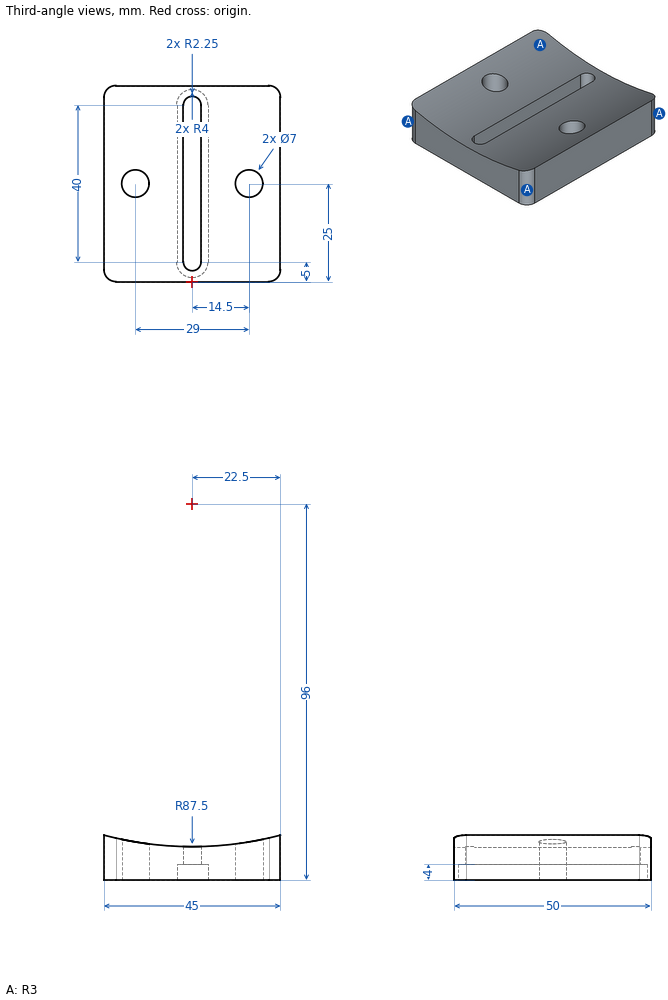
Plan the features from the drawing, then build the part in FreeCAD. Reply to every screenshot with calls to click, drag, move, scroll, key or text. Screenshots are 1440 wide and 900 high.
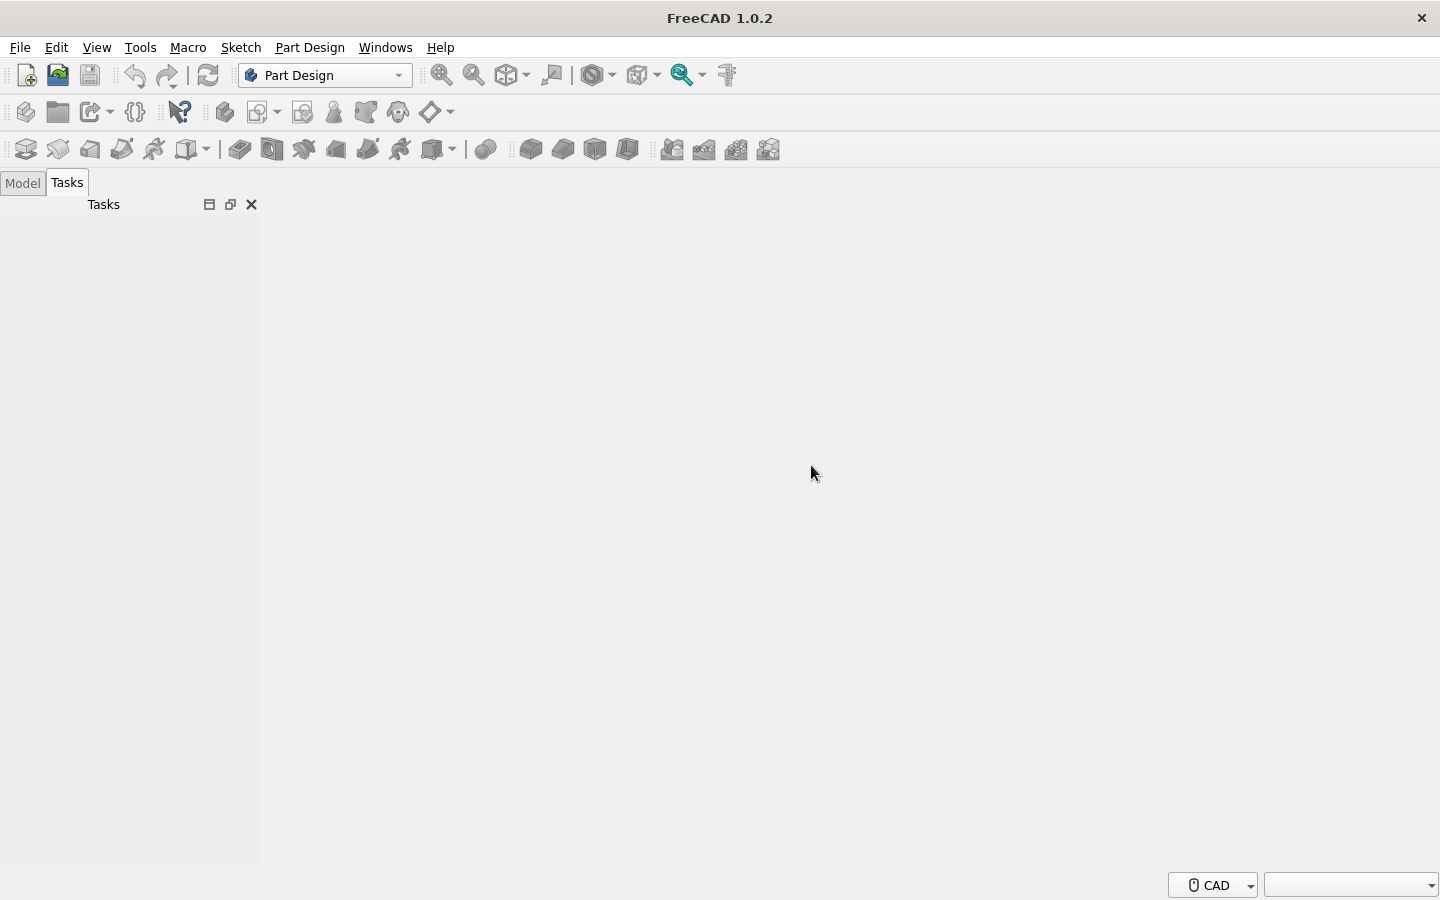
click(26, 76)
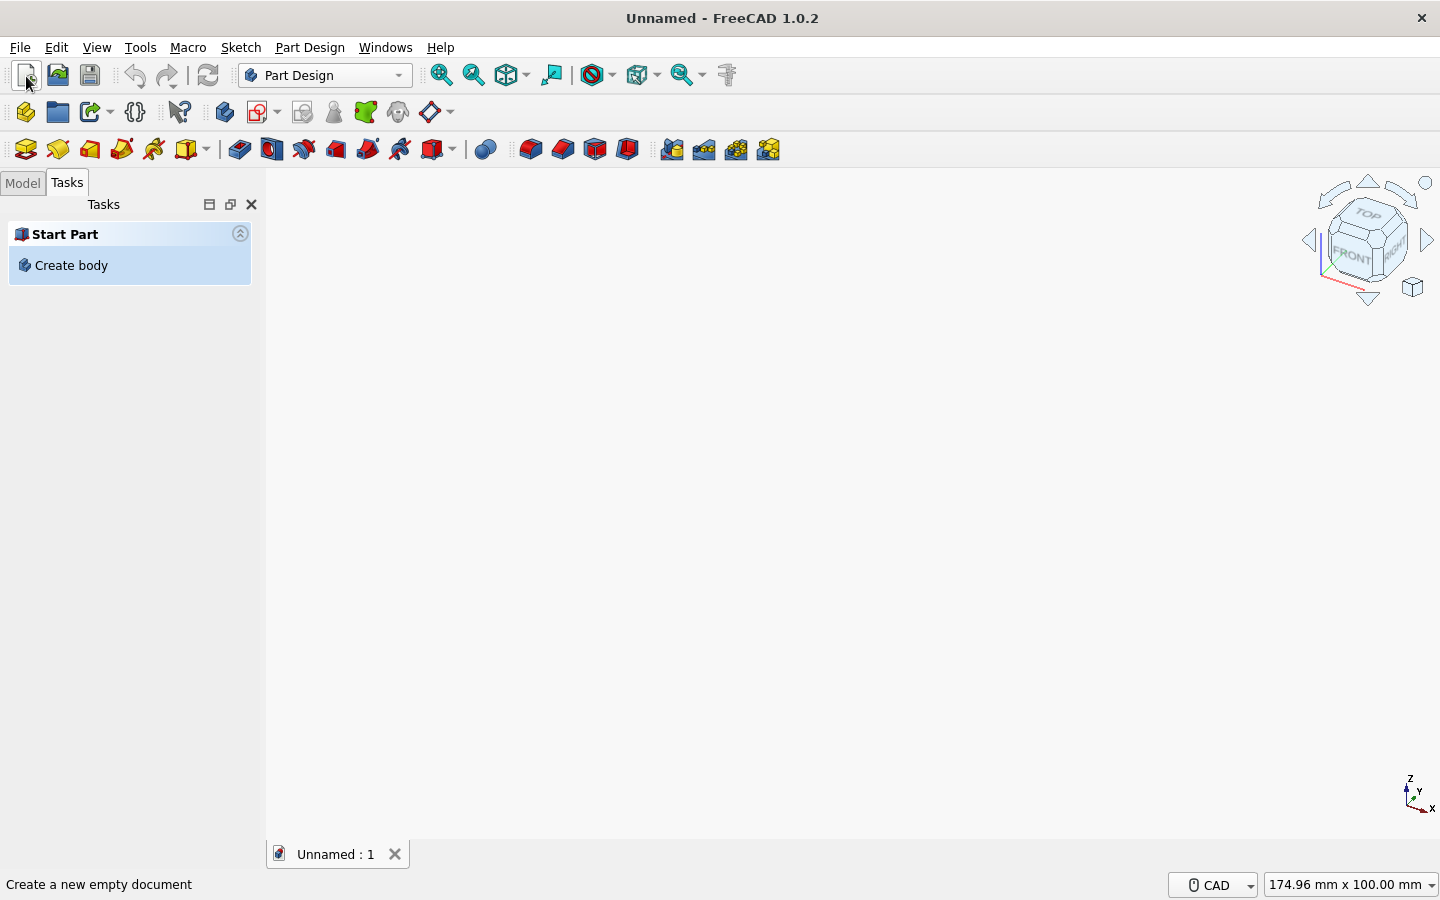
click(258, 112)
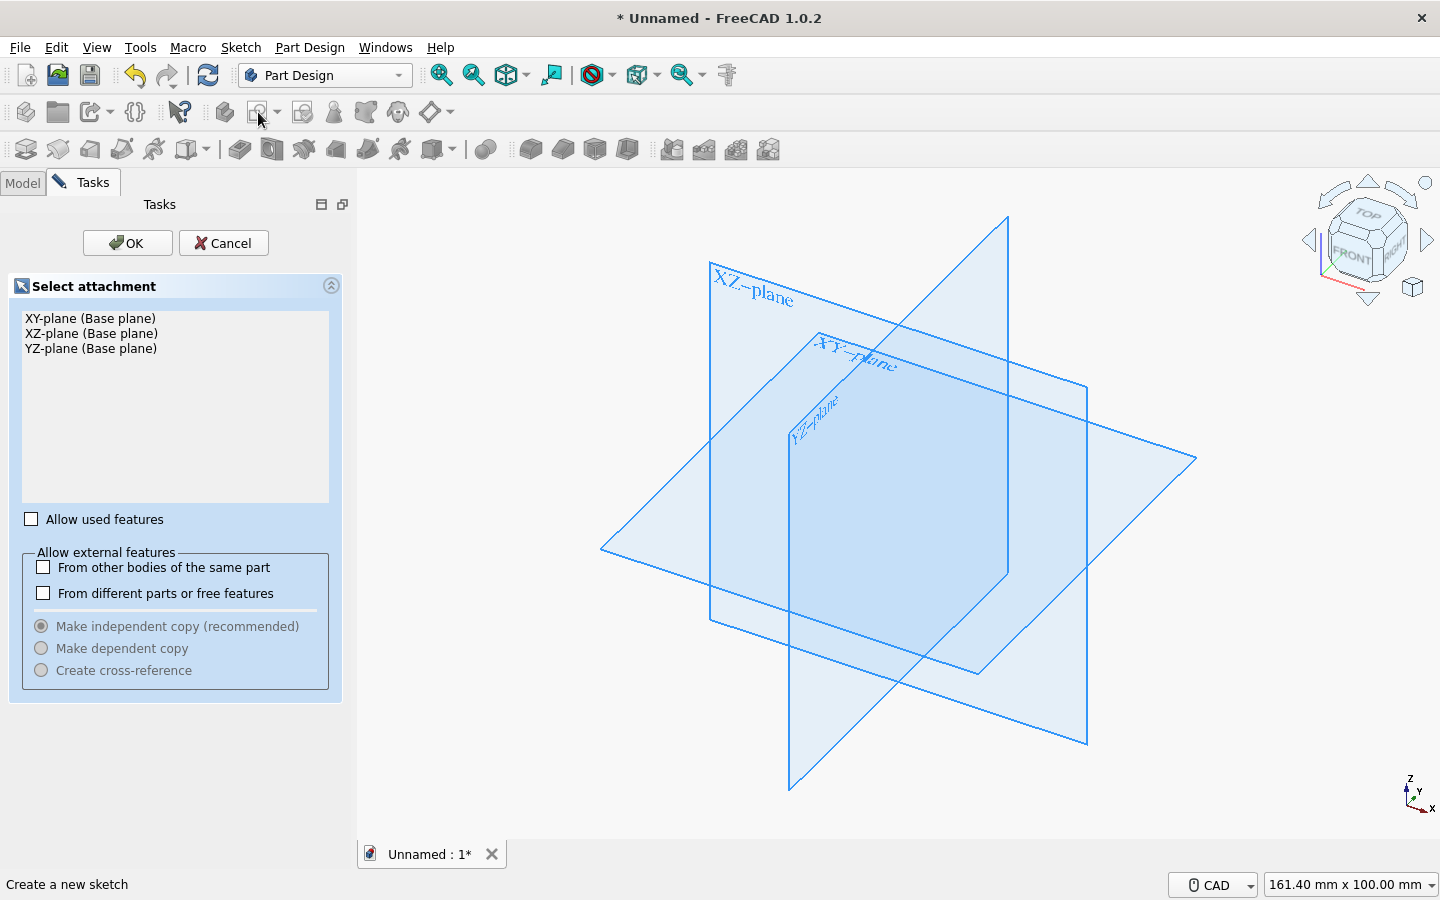
click(82, 334)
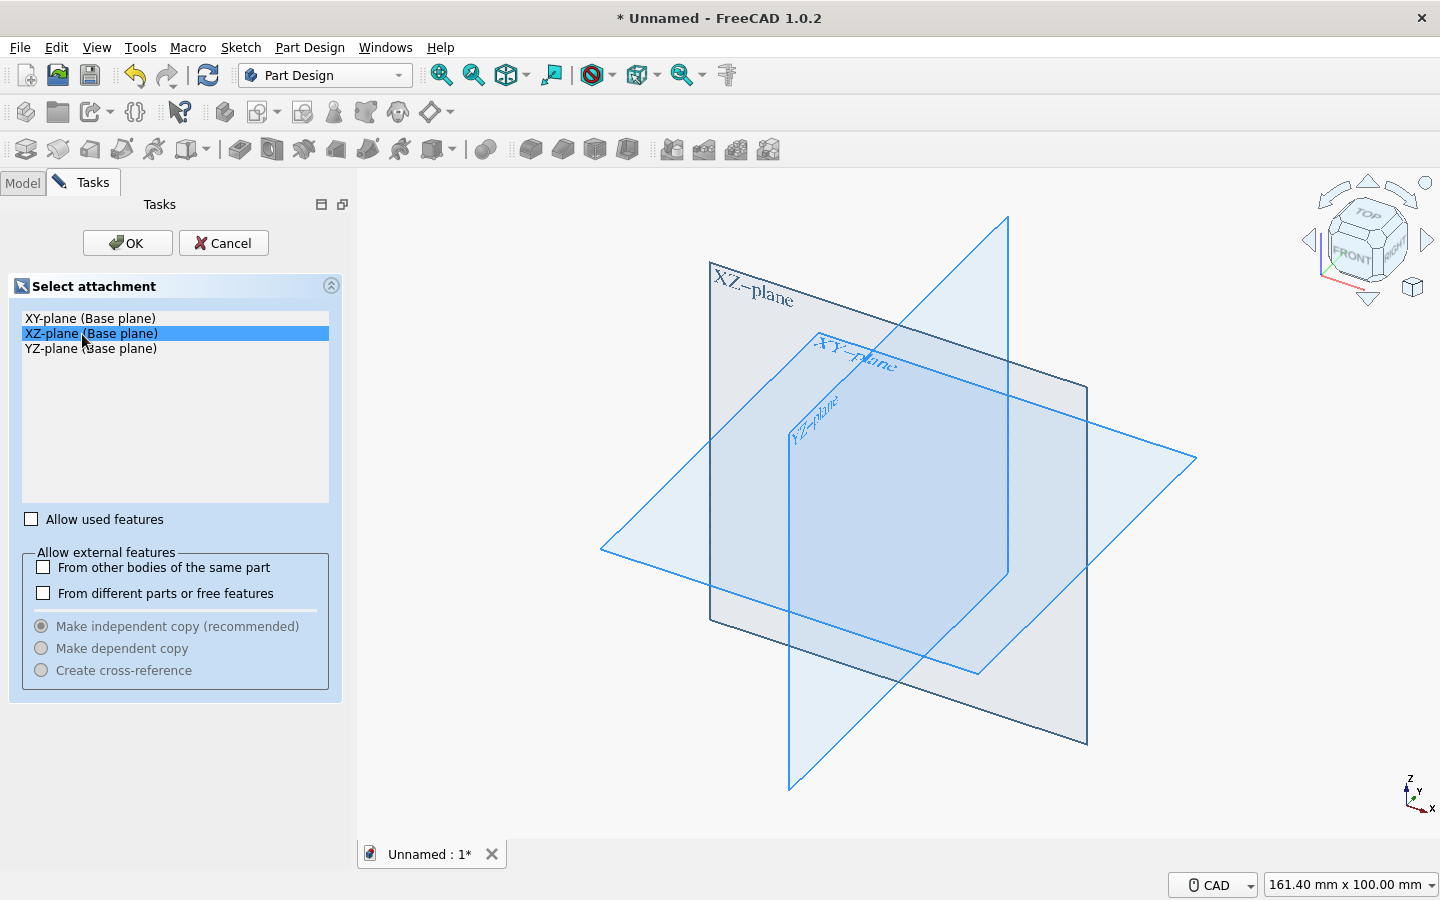
click(128, 243)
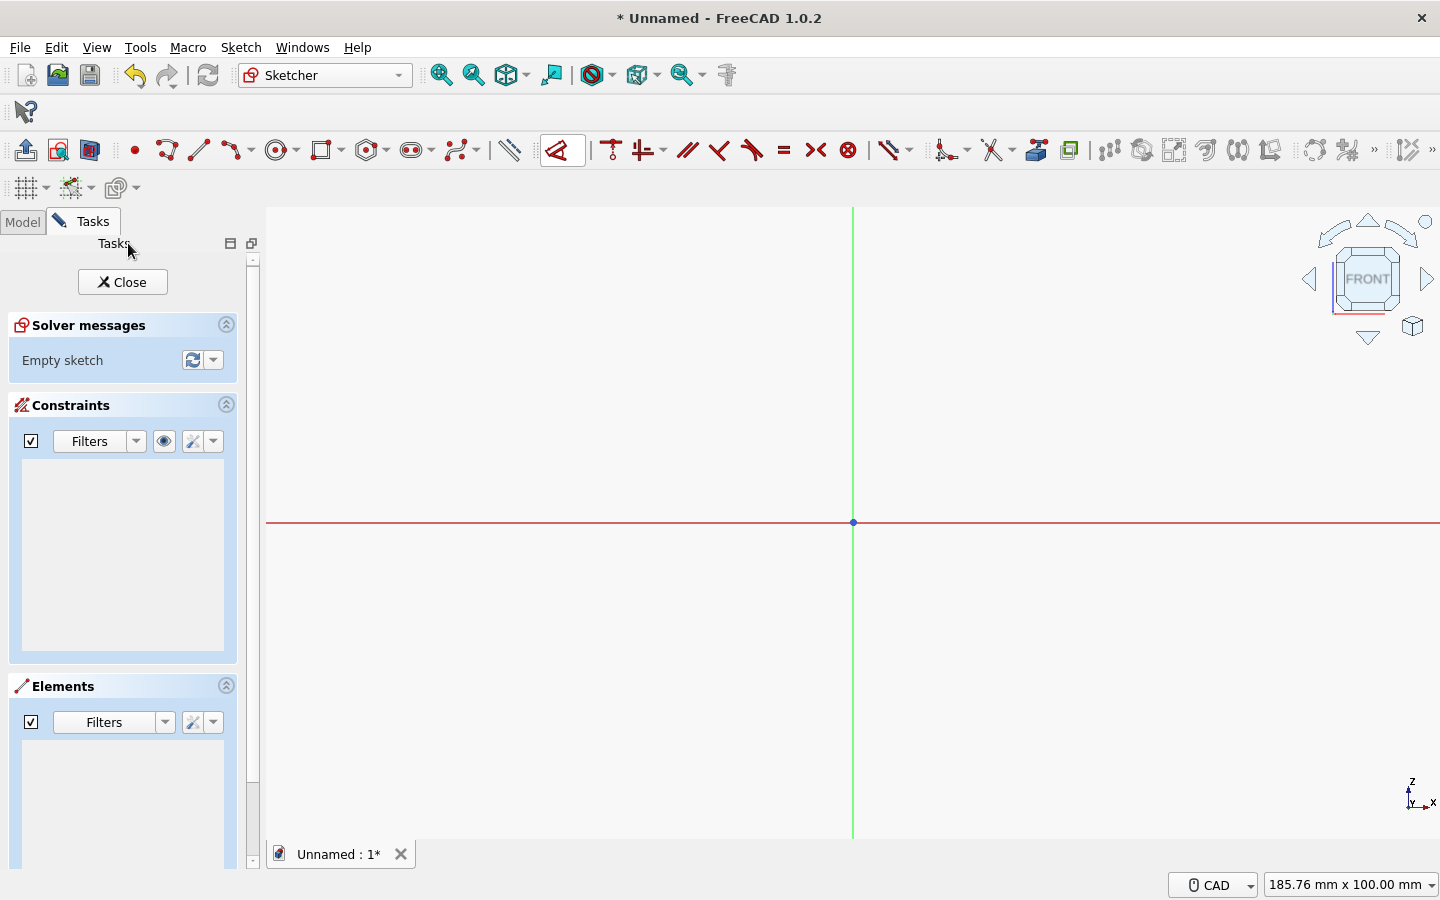
scroll(701, 235, down, 3)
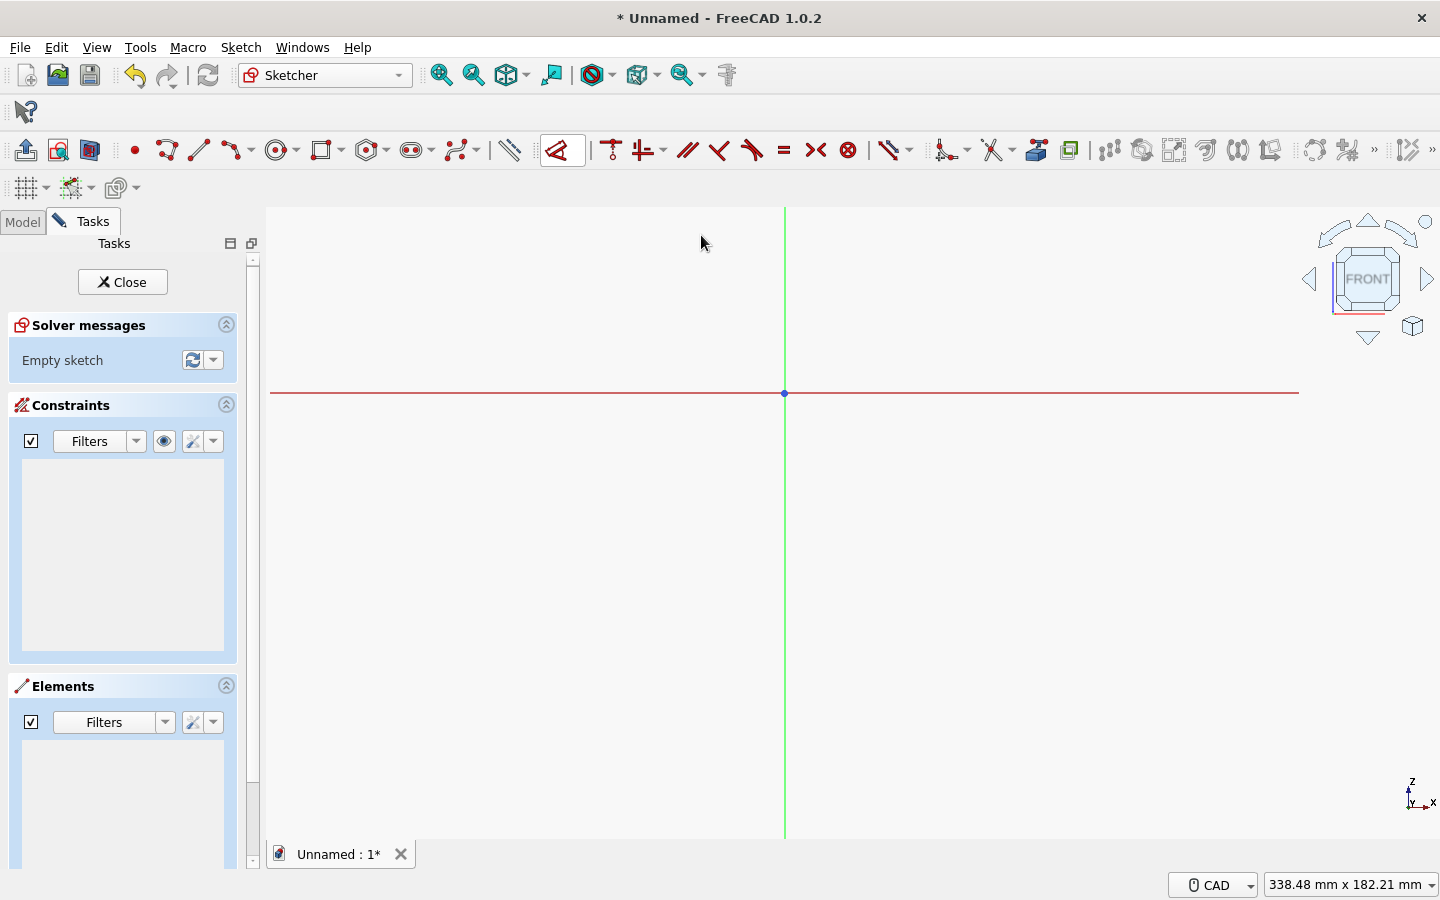
click(168, 150)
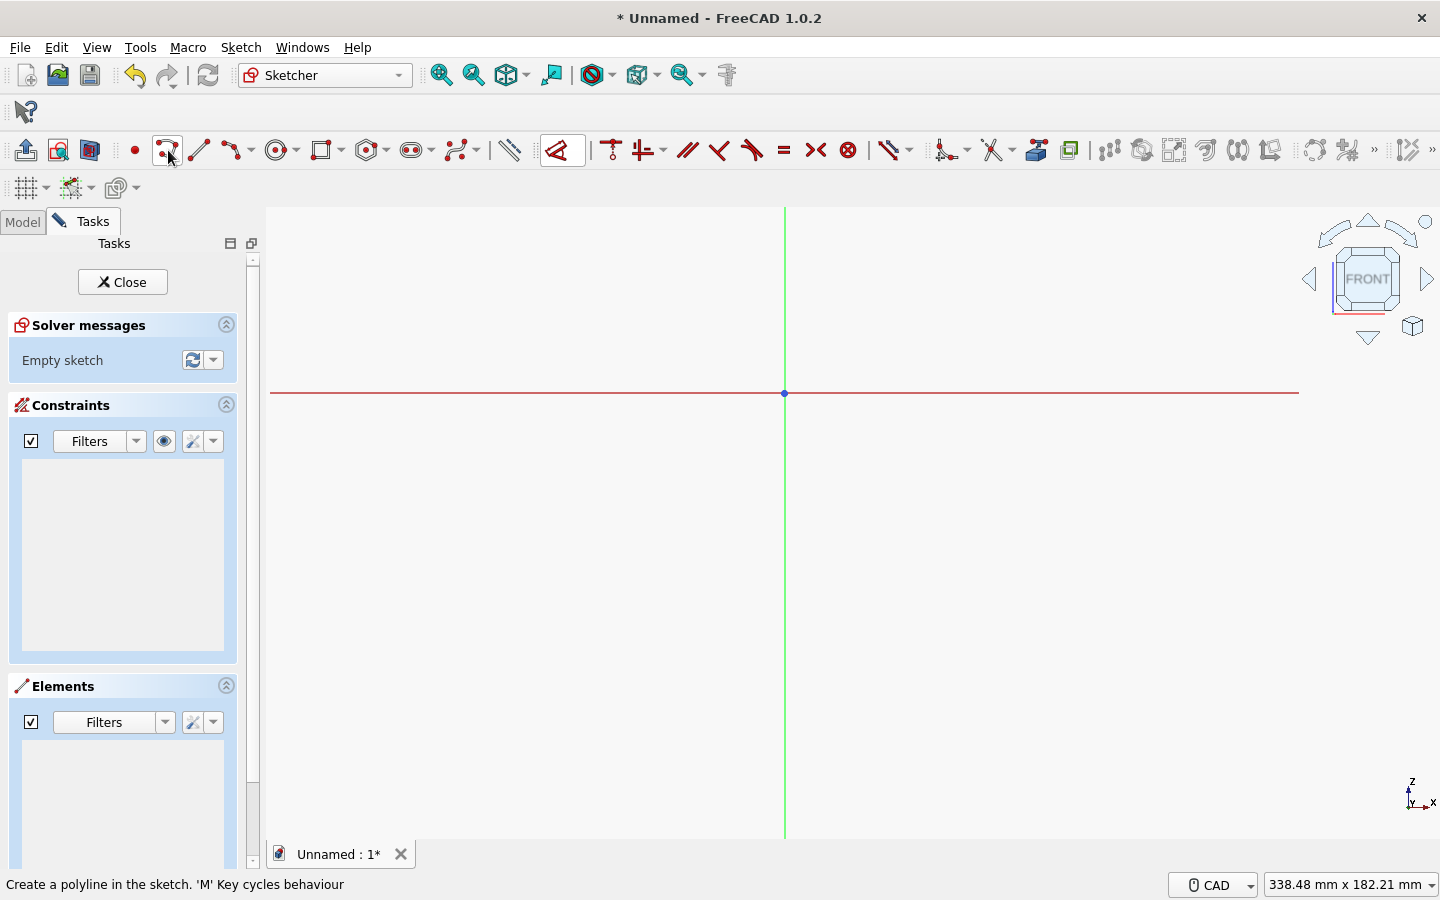
click(863, 686)
click(863, 726)
click(707, 726)
click(707, 686)
right_click(707, 686)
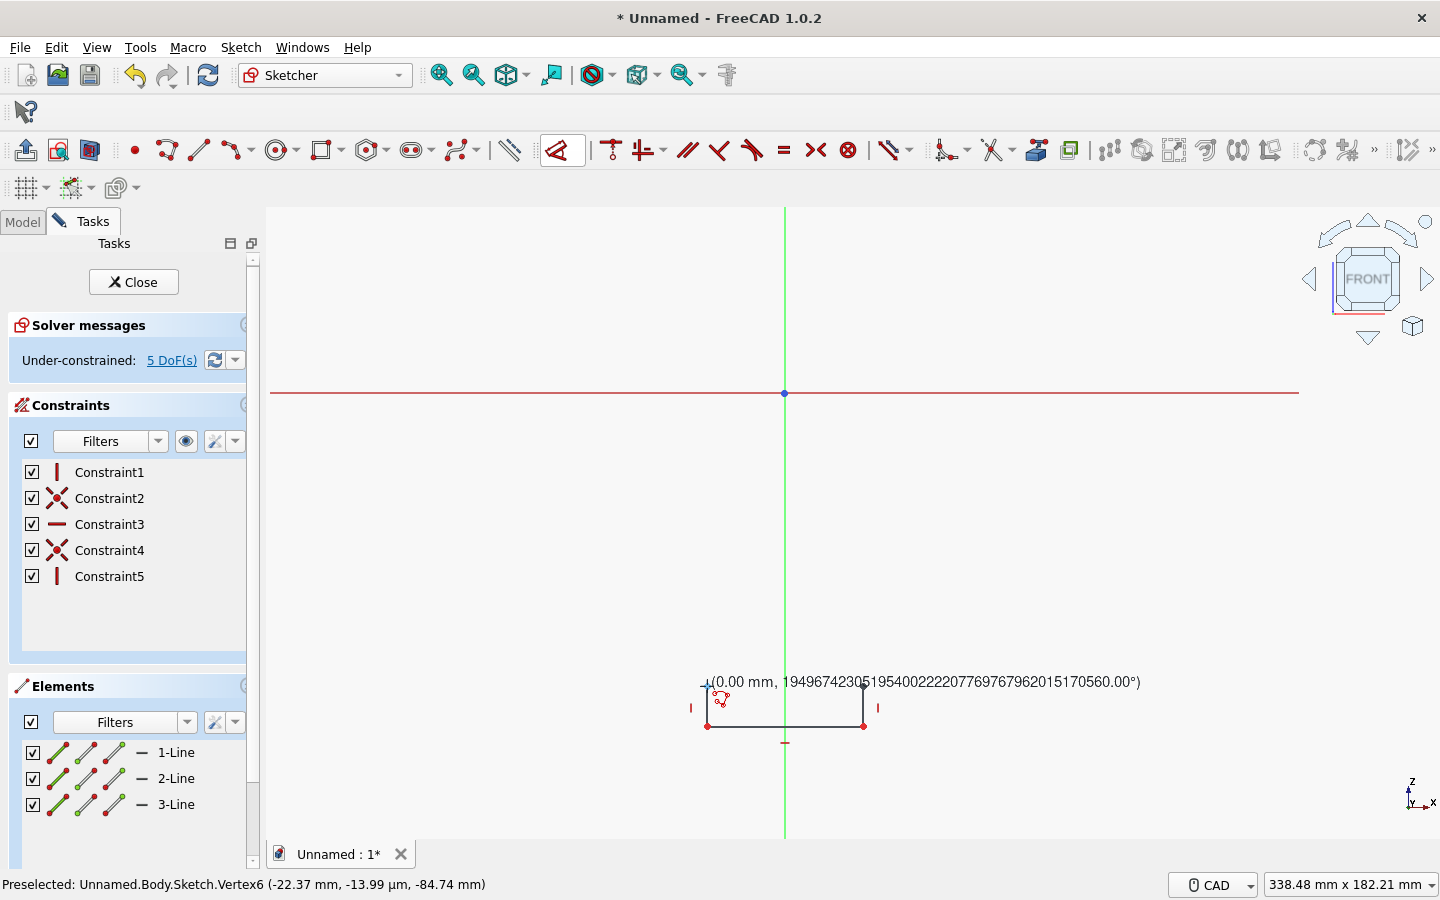
click(232, 150)